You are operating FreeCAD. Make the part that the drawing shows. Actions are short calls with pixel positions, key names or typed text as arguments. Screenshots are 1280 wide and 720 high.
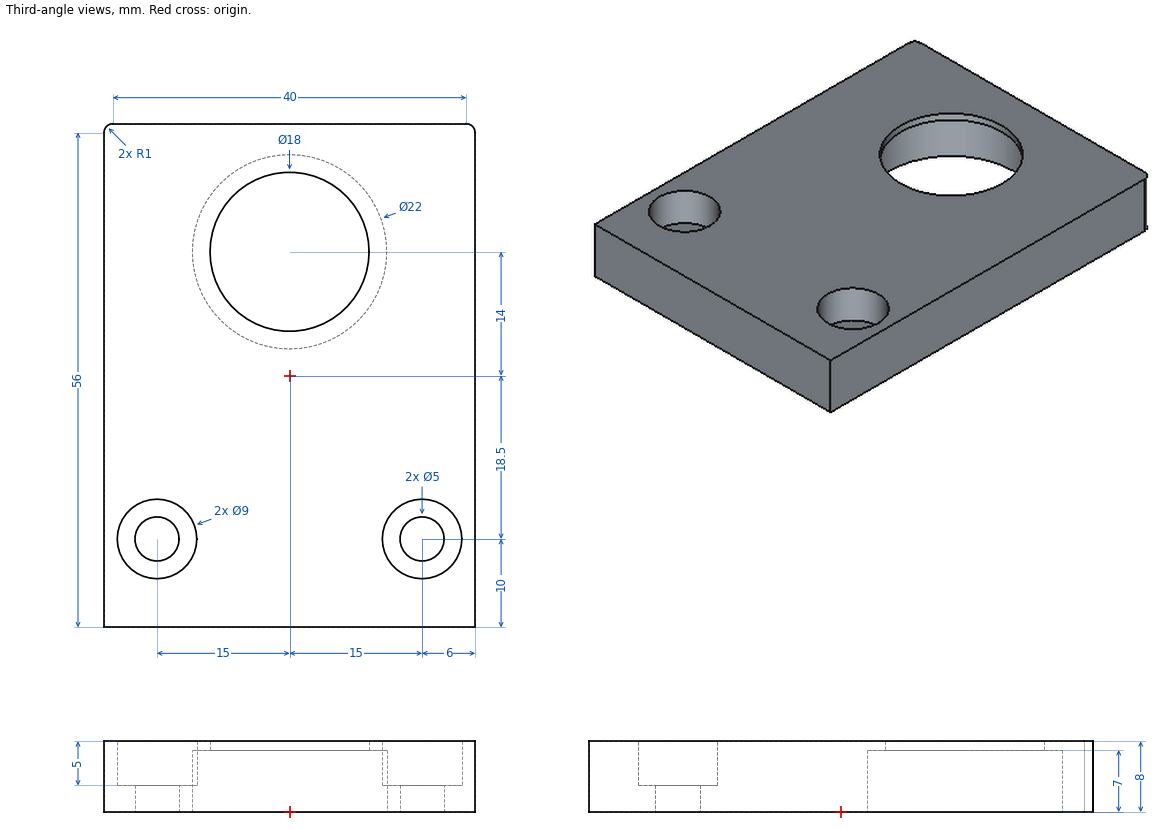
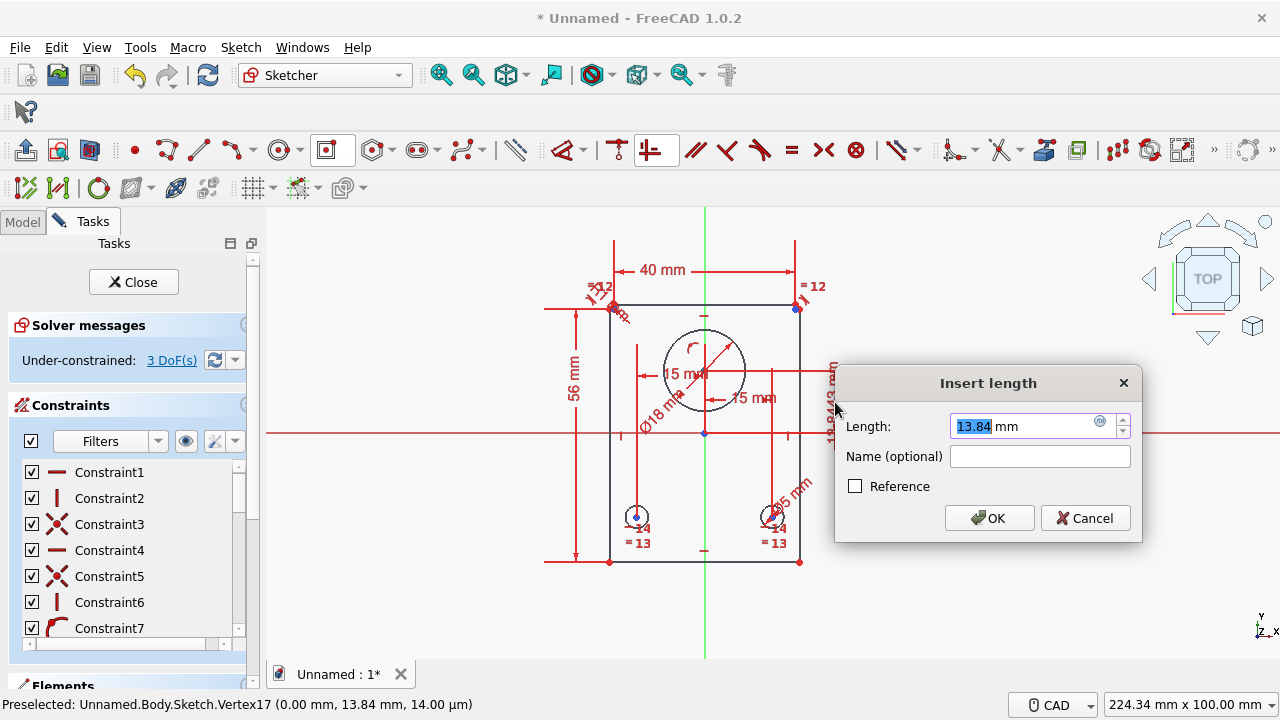
text(14)
key(Return)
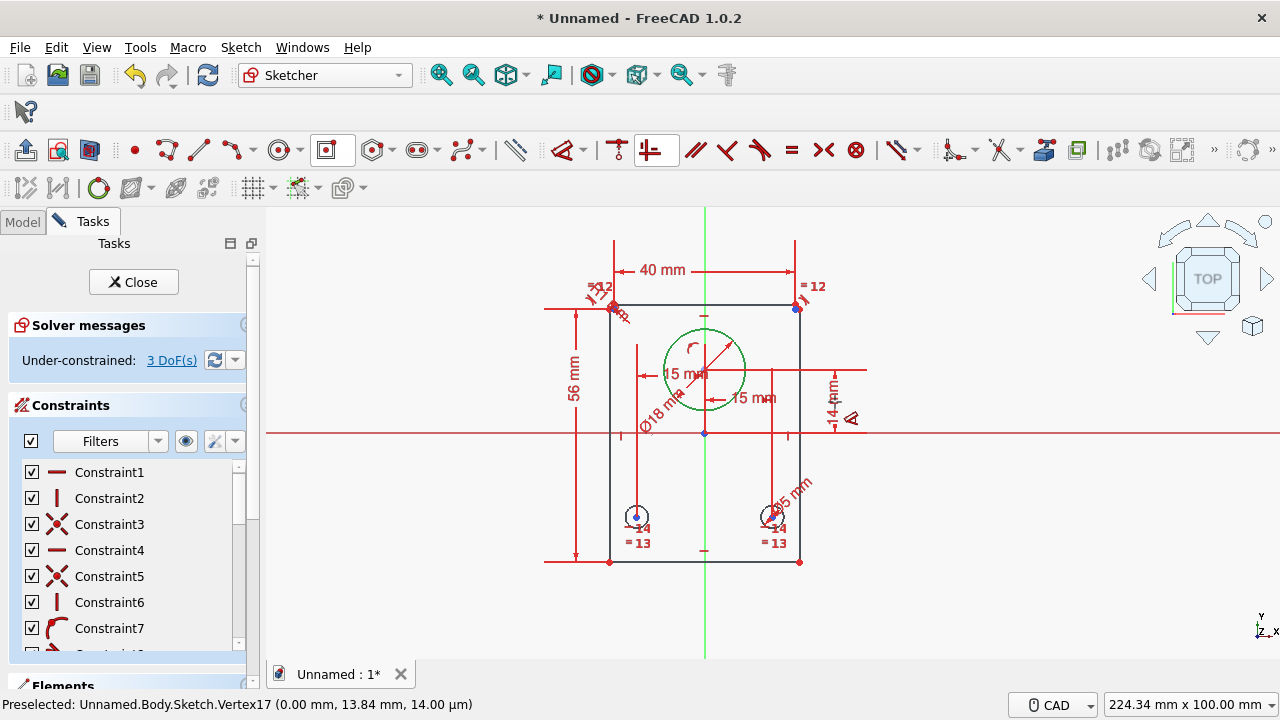
scroll(800, 562, up, 2)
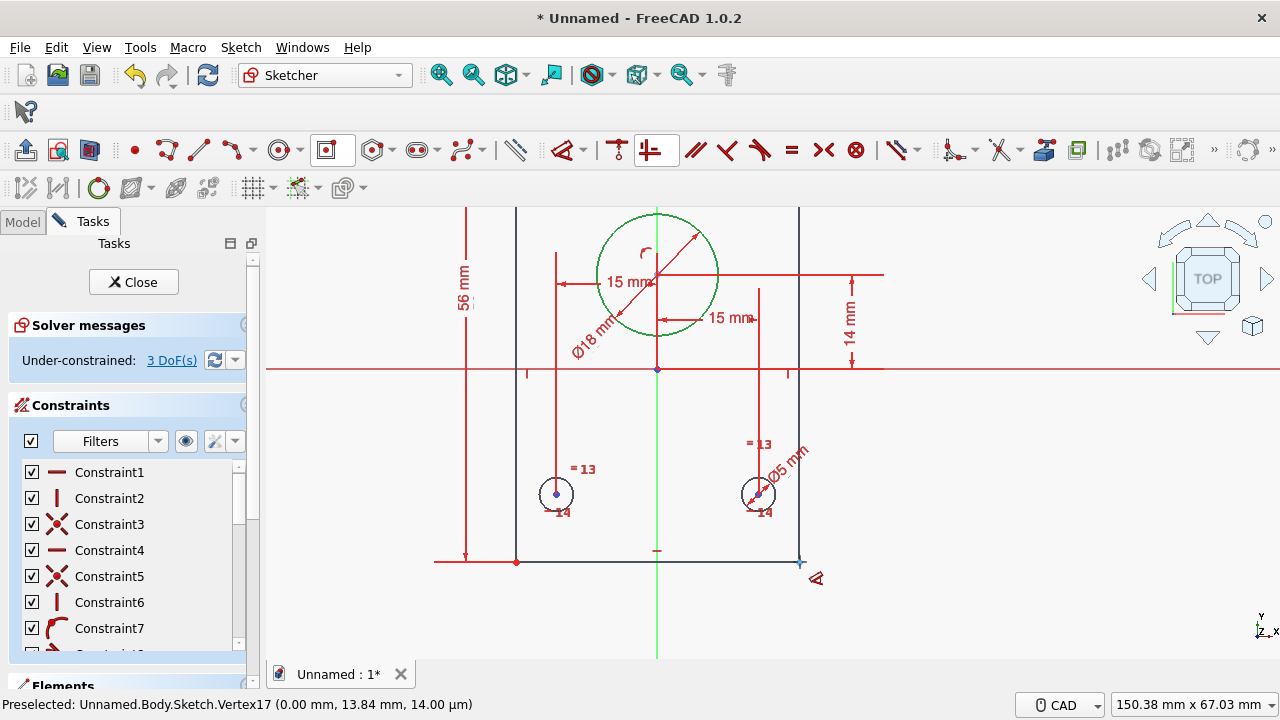
click(799, 562)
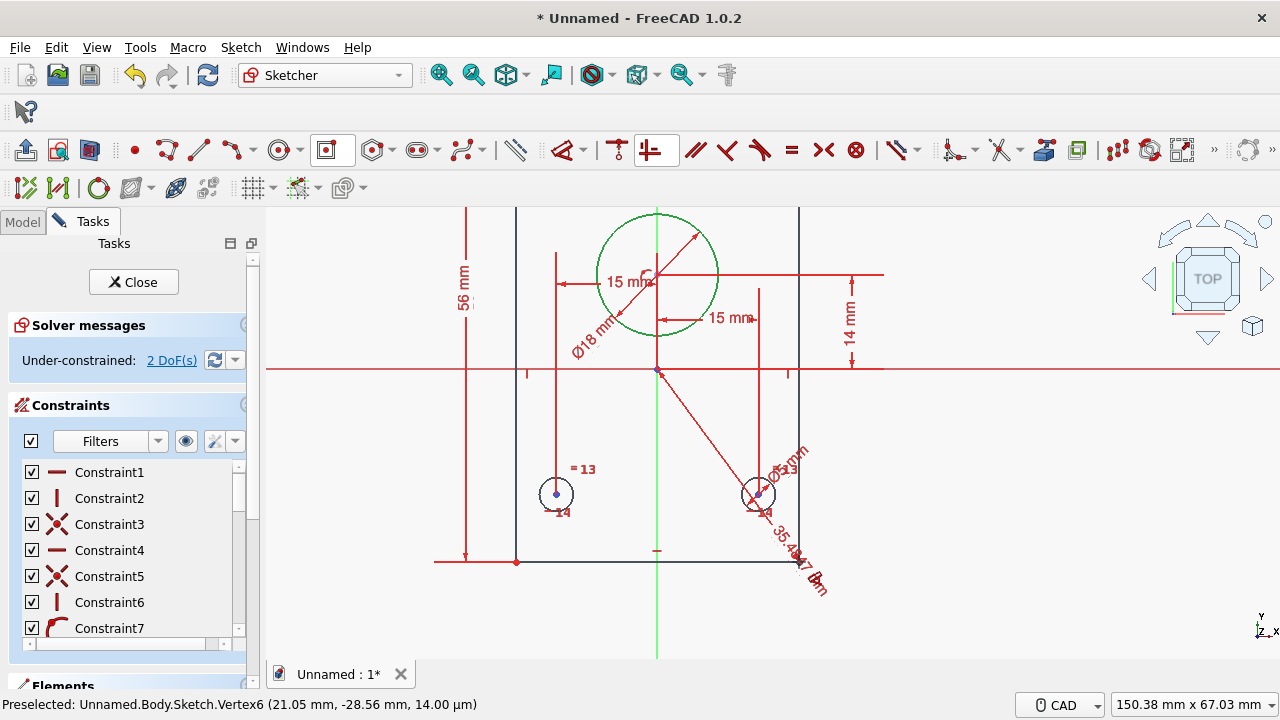
click(759, 495)
click(779, 596)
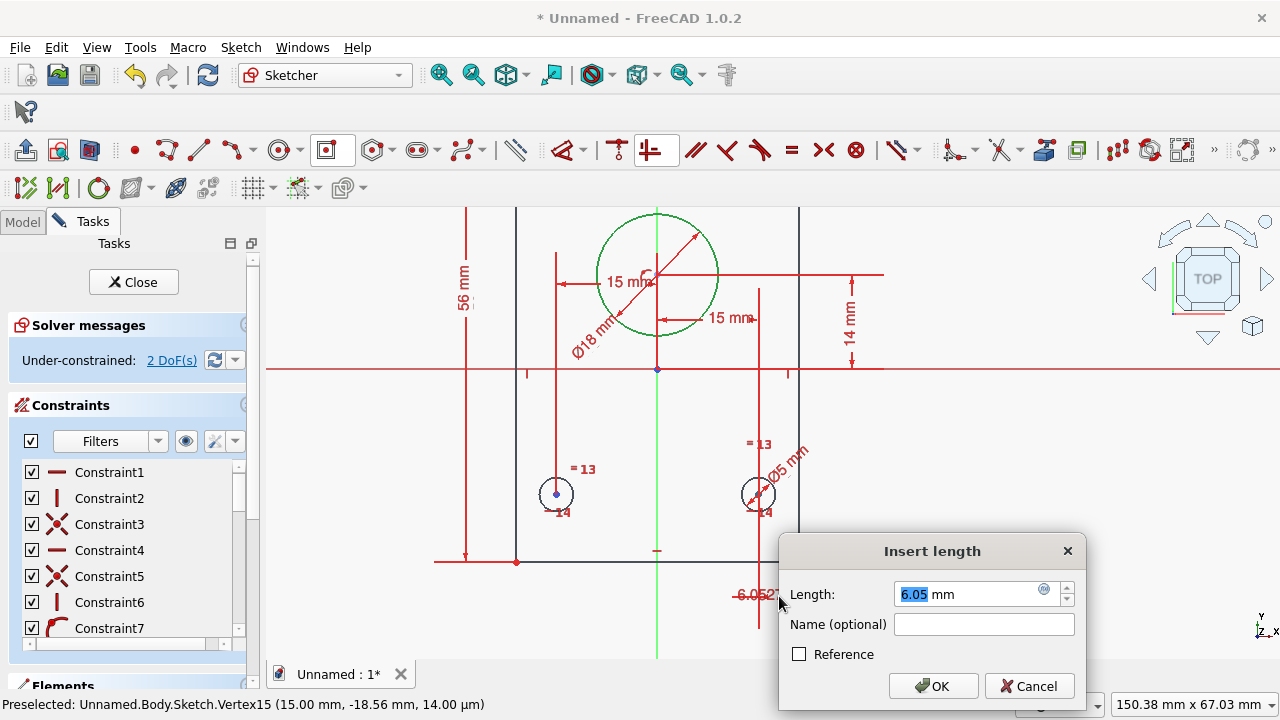
text(6)
key(Return)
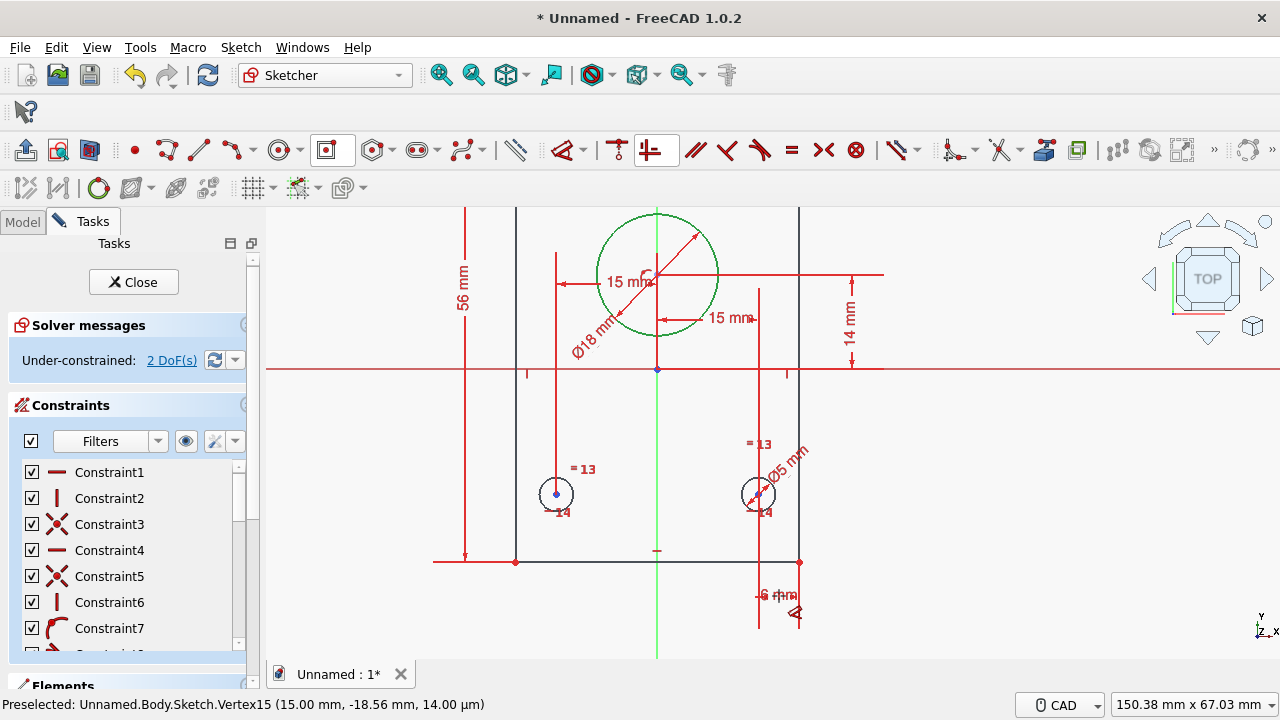
click(799, 562)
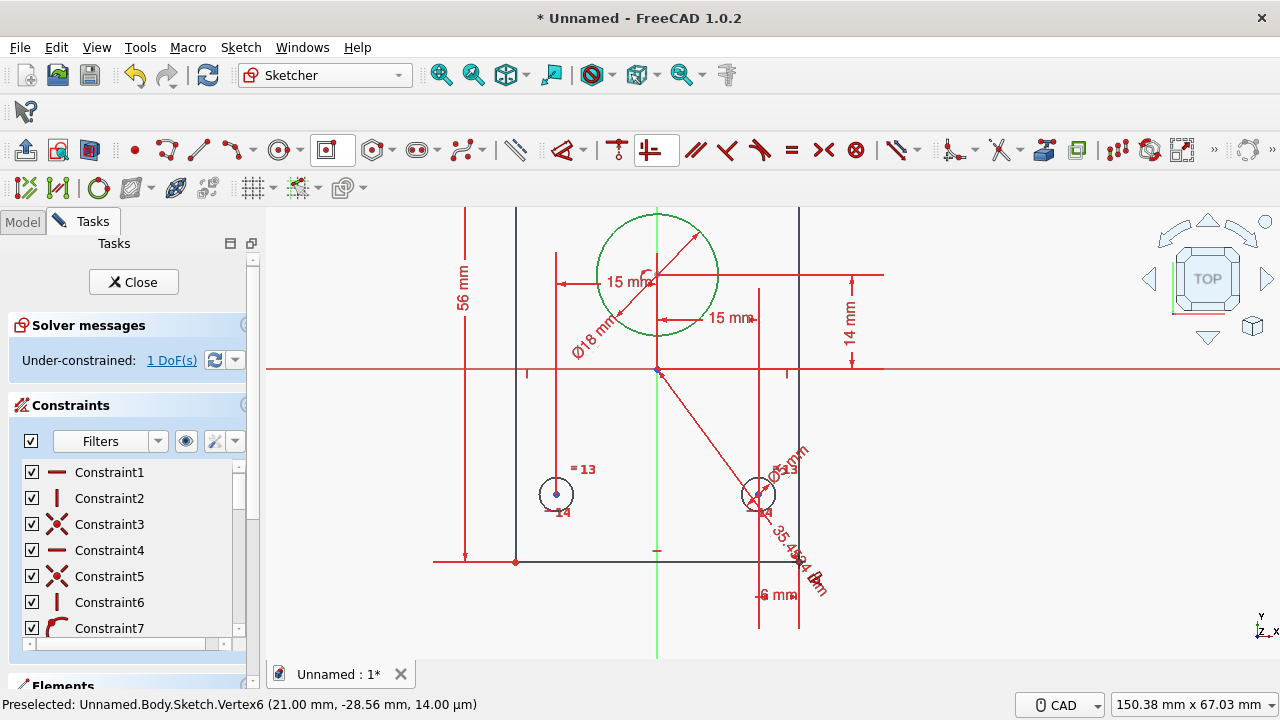
click(759, 495)
click(833, 528)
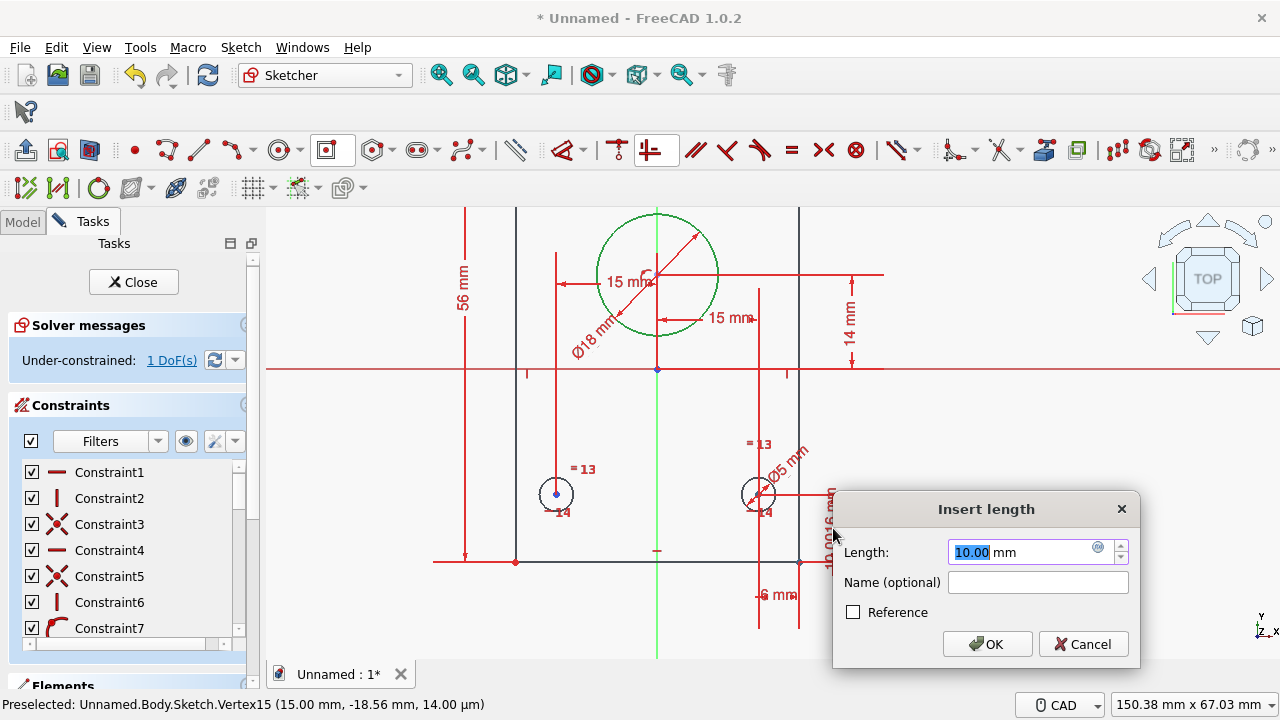
text(10)
key(Return)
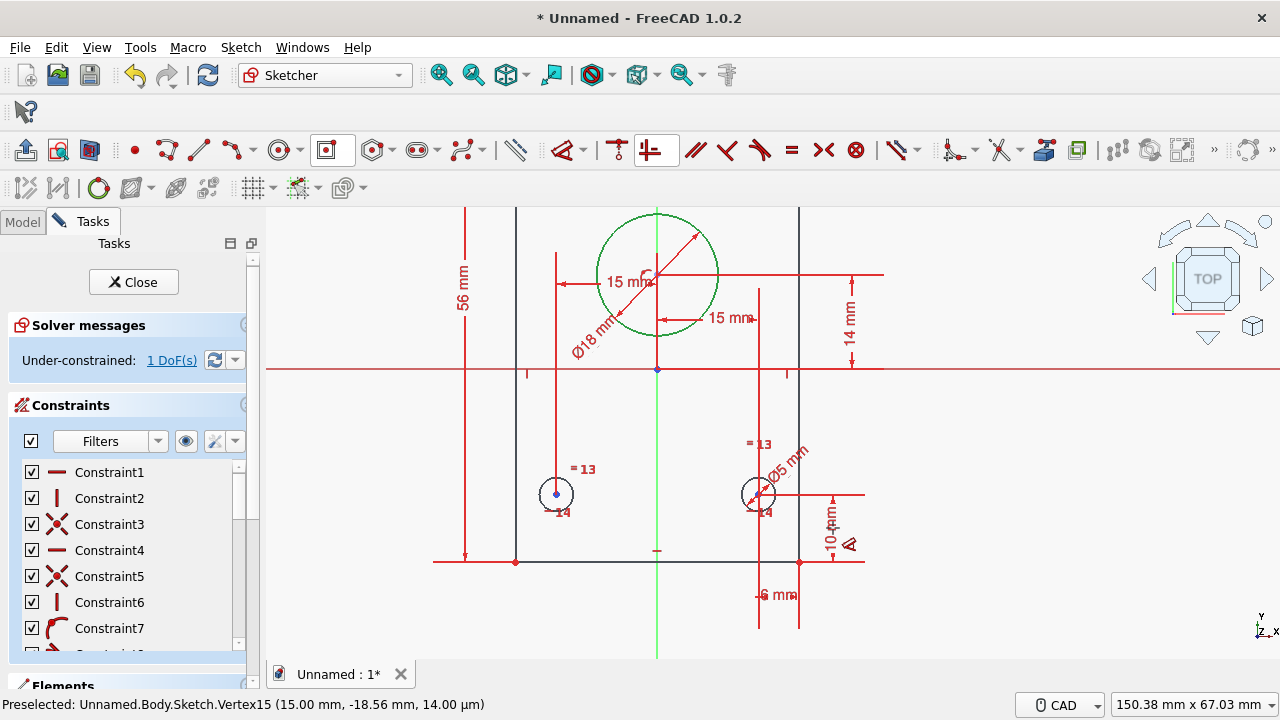
click(759, 495)
click(623, 432)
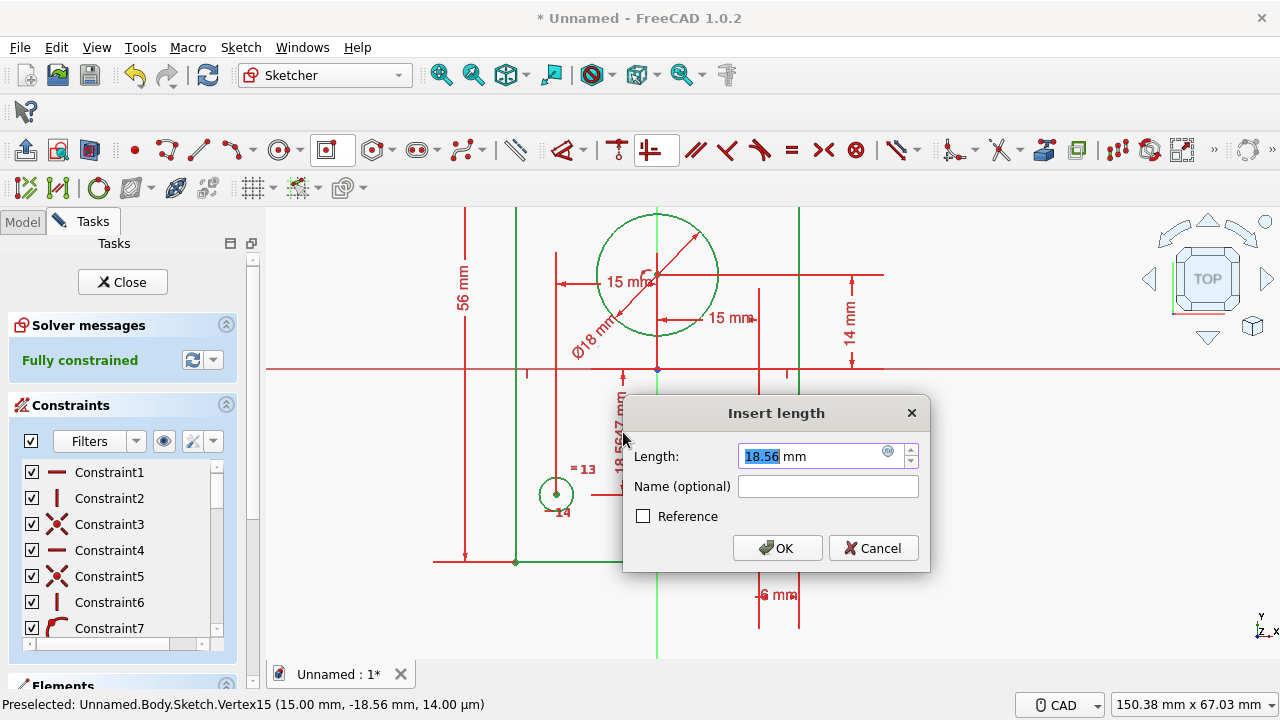
text(18.5)
key(Return)
key(Escape)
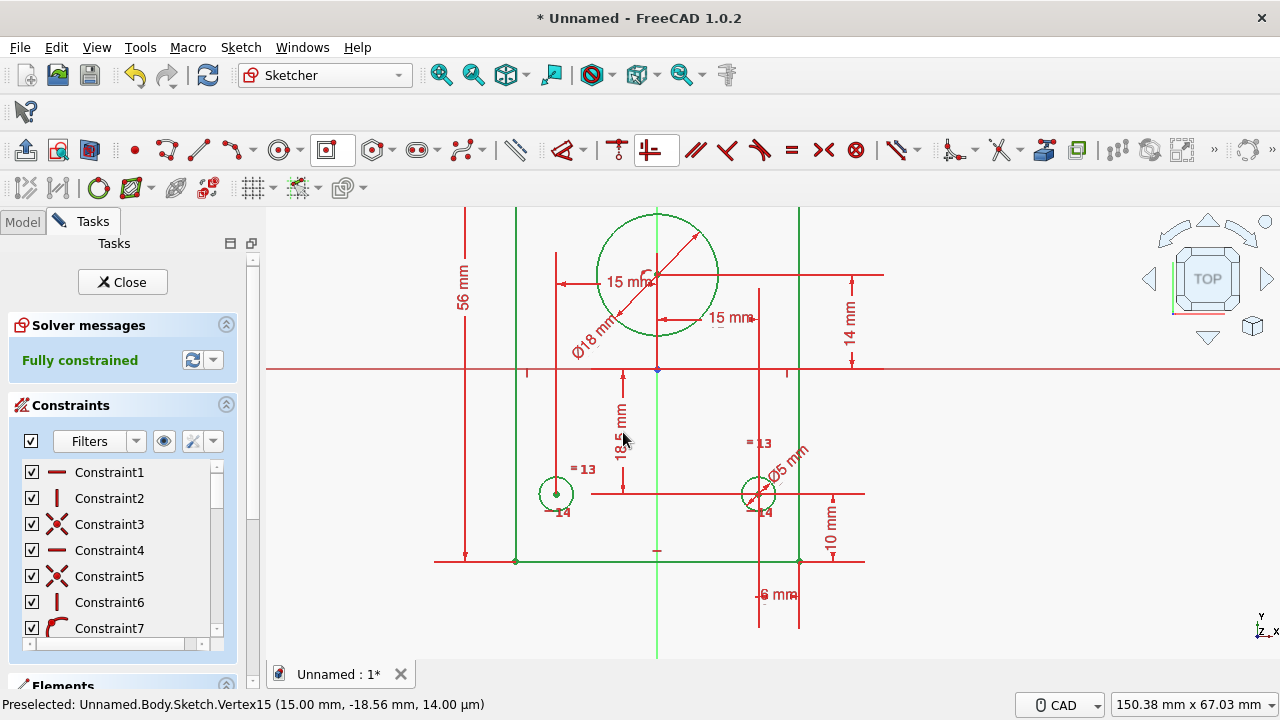
click(123, 282)